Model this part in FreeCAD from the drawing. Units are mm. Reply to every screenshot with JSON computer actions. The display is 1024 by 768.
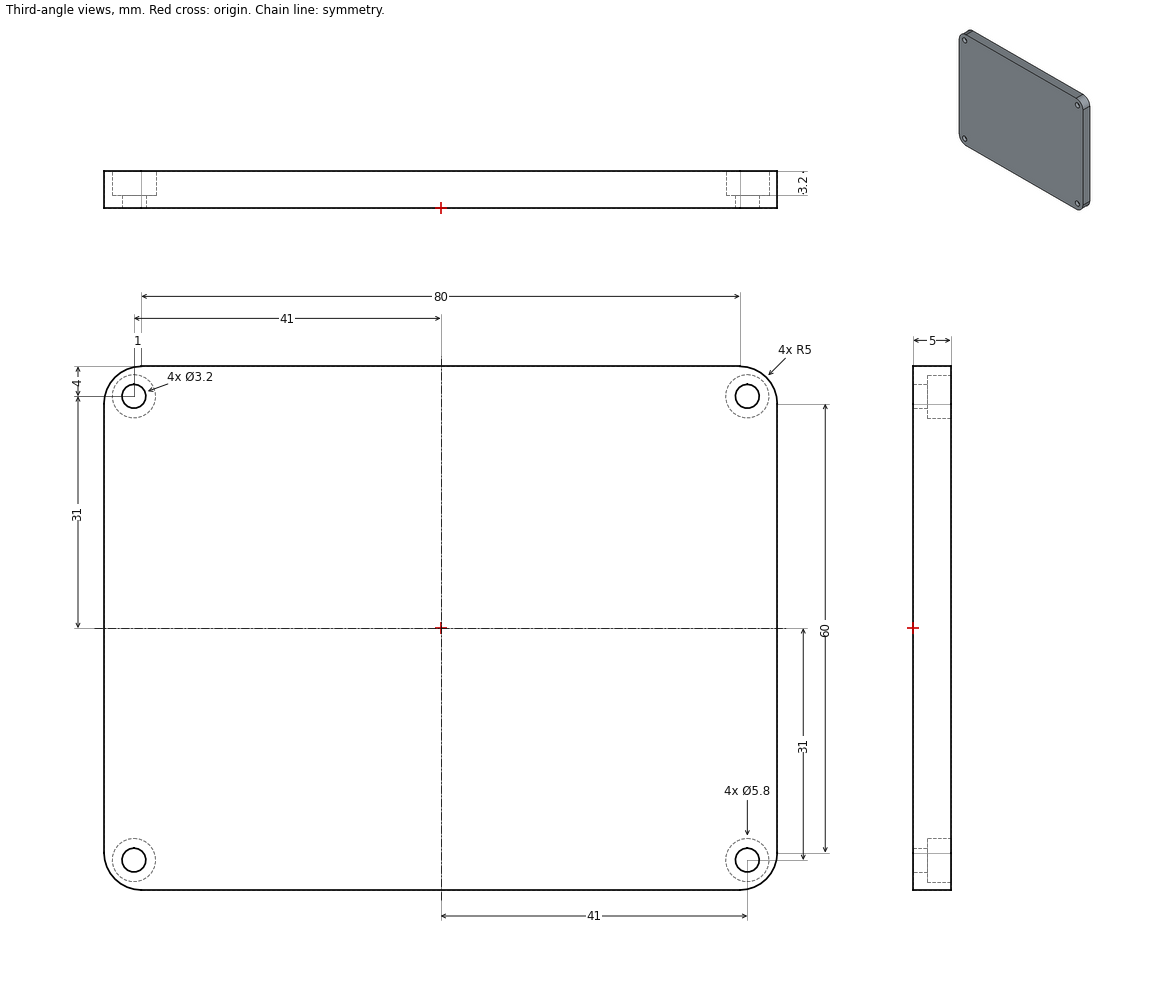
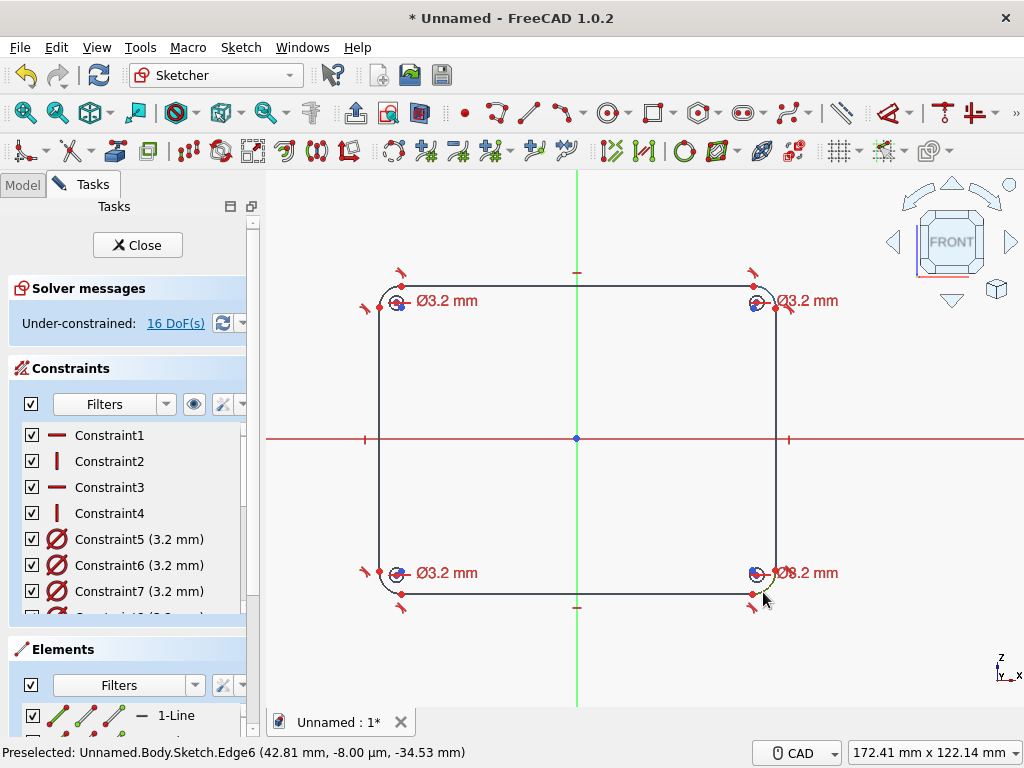
{"action": "scroll", "coordinate": [382, 582], "scroll_direction": "up", "scroll_amount": 3}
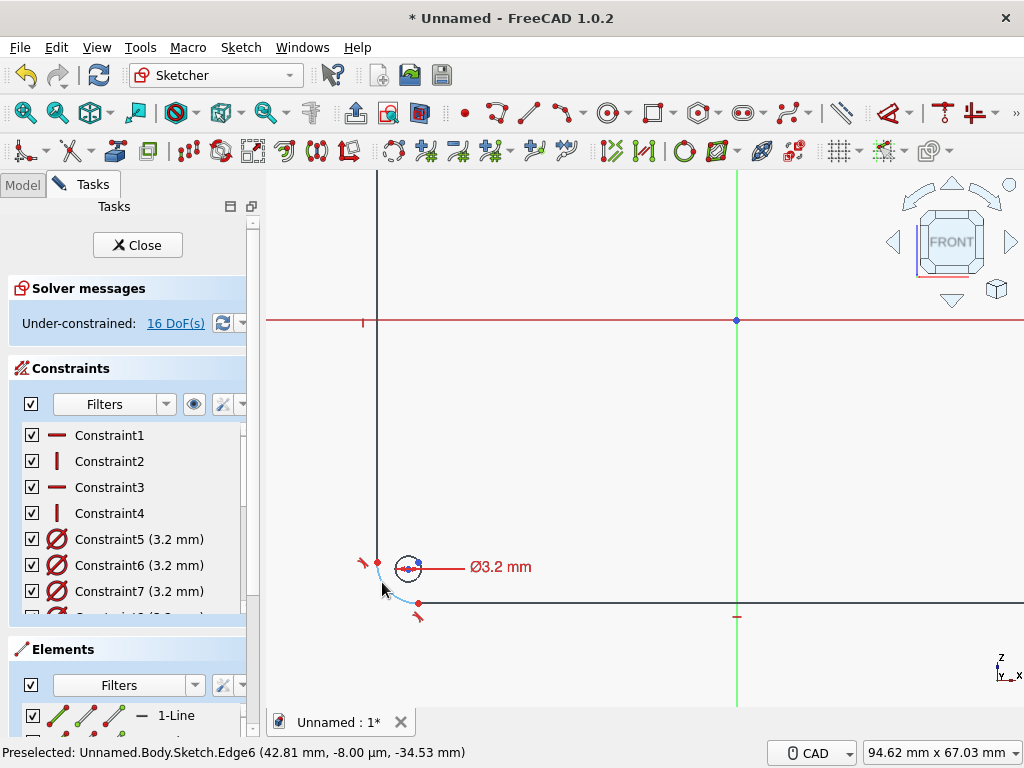
{"action": "left_click", "coordinate": [382, 581]}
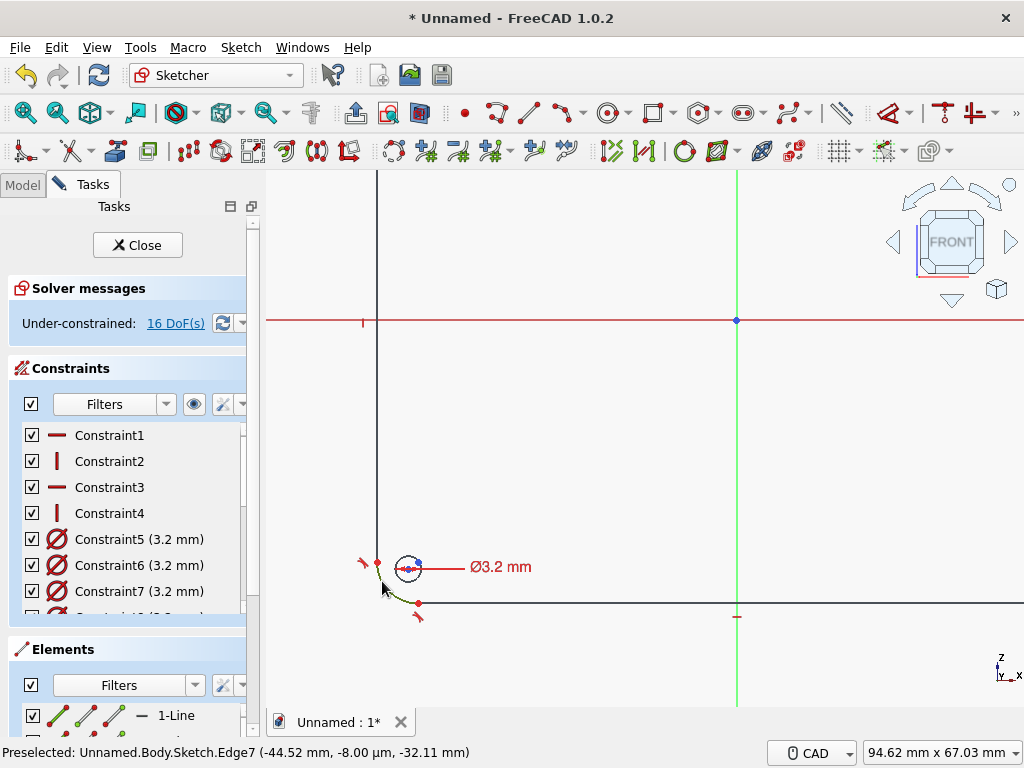
{"action": "scroll", "coordinate": [382, 582], "scroll_direction": "down", "scroll_amount": 3}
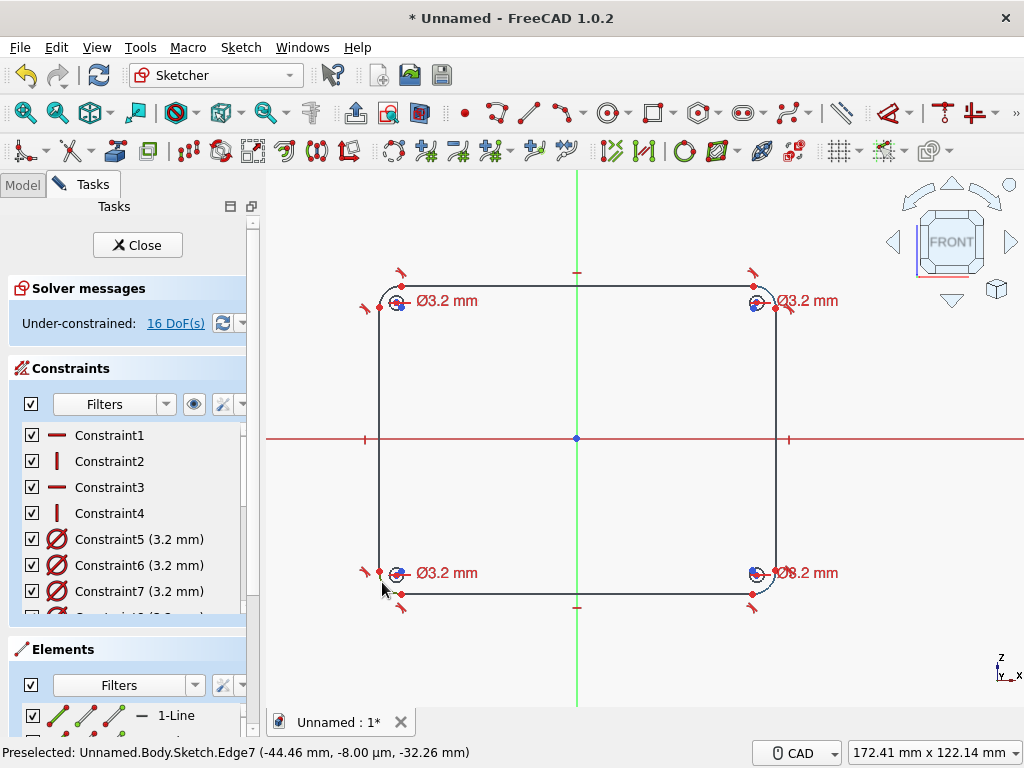
{"action": "scroll", "coordinate": [391, 288], "scroll_direction": "up", "scroll_amount": 3}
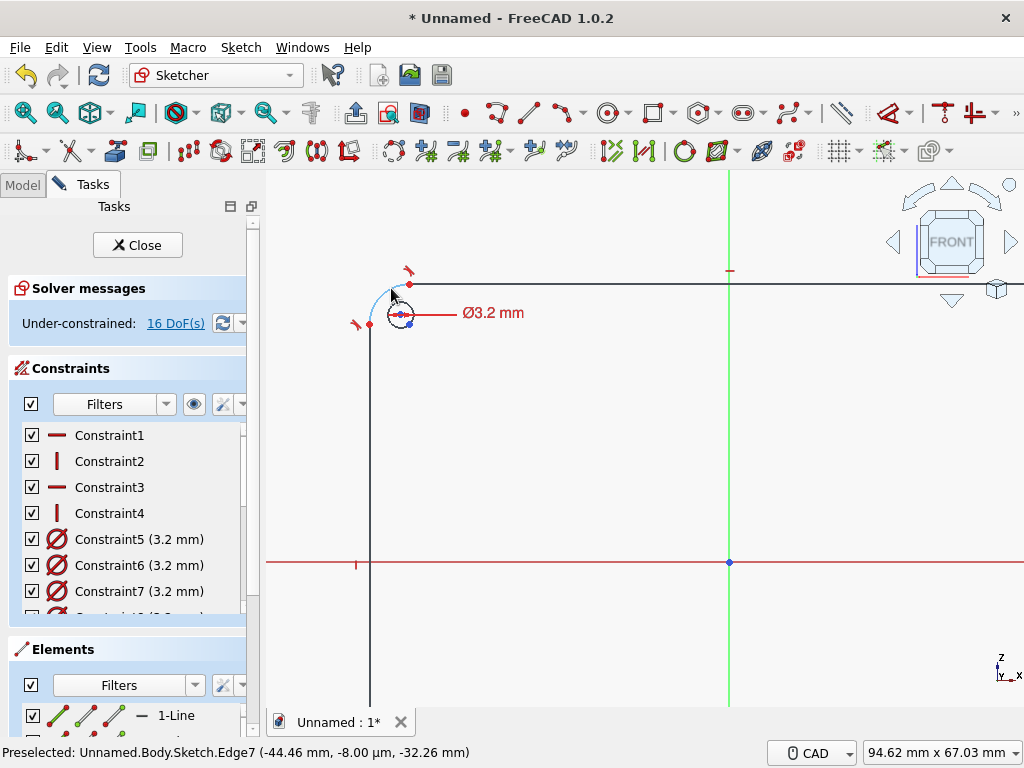
{"action": "left_click", "coordinate": [392, 289]}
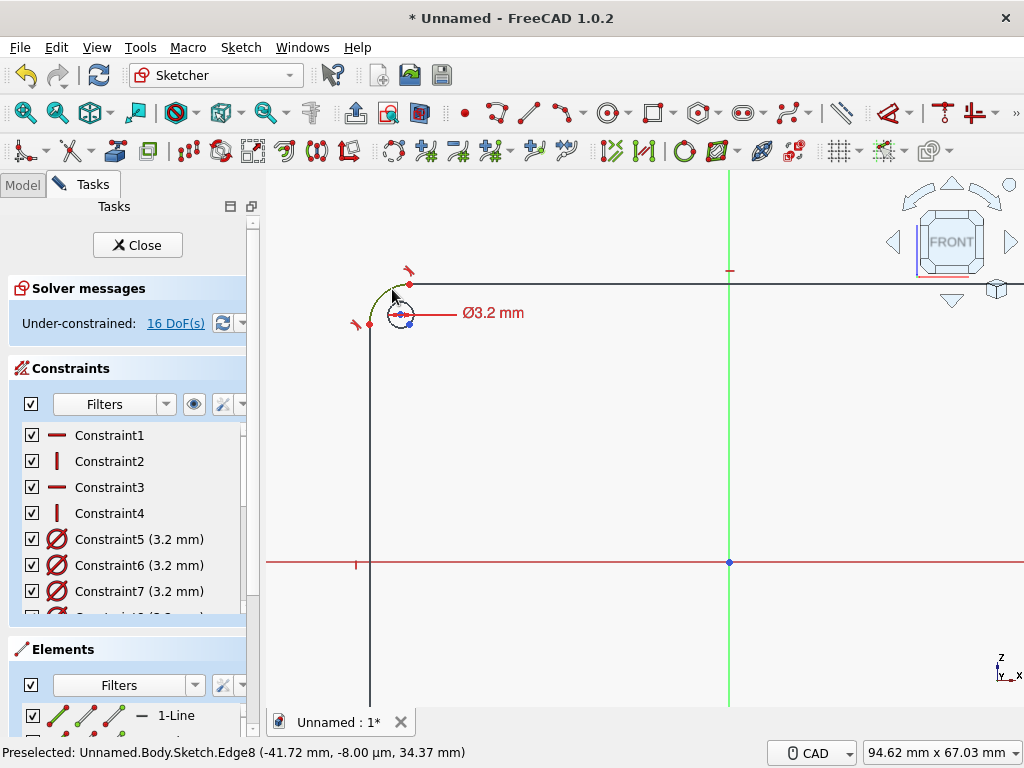
{"action": "key", "text": "e"}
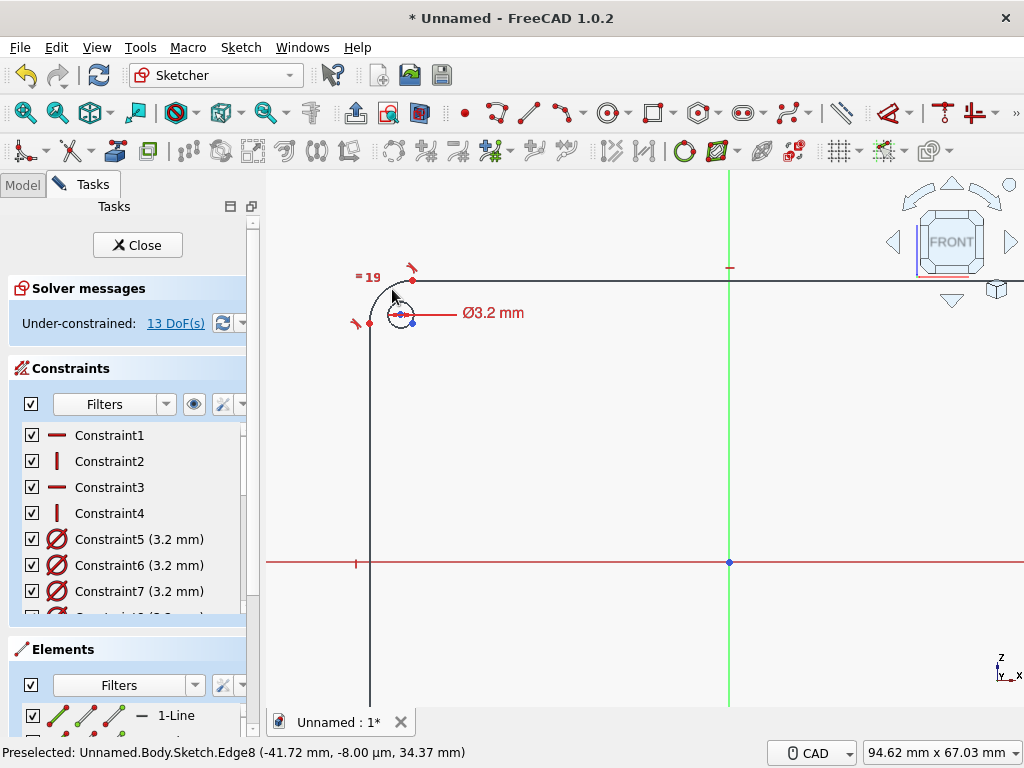
{"action": "left_click", "coordinate": [401, 315]}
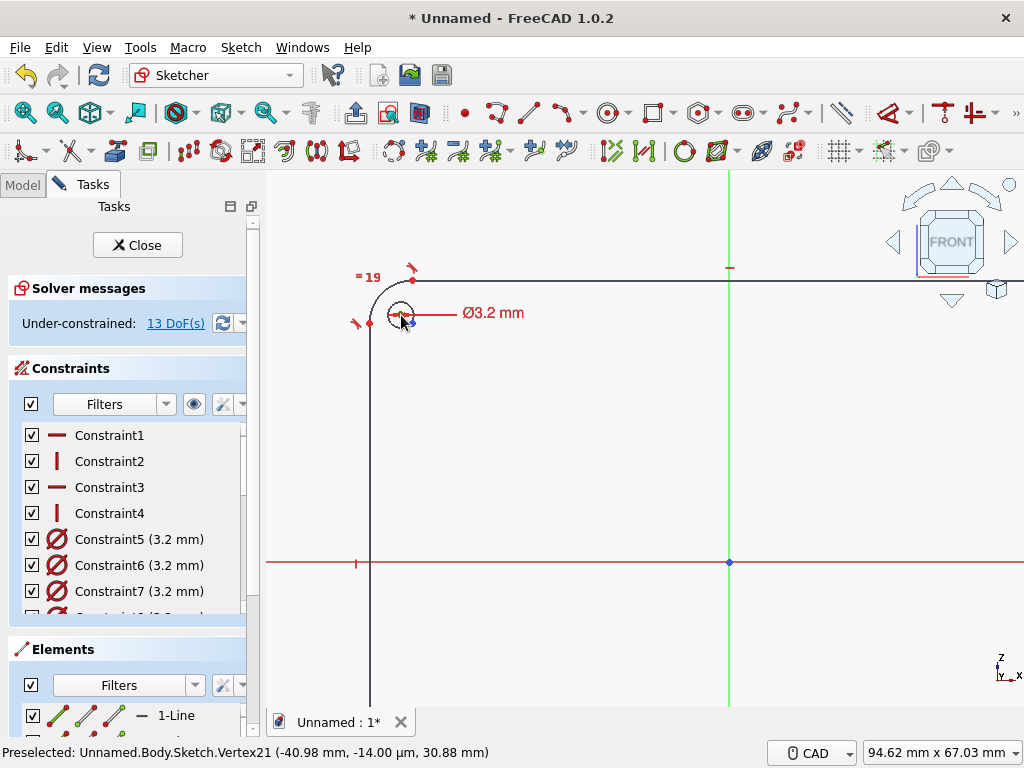
{"action": "scroll", "coordinate": [391, 288], "scroll_direction": "down", "scroll_amount": 3}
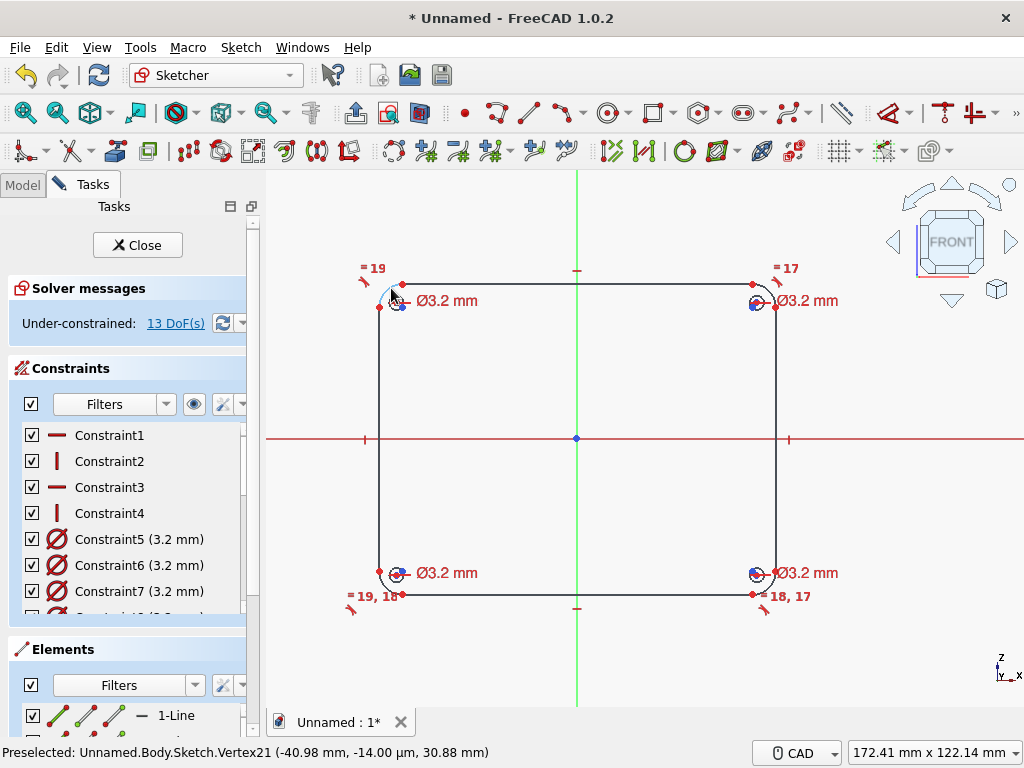
{"action": "scroll", "coordinate": [757, 303], "scroll_direction": "up", "scroll_amount": 4}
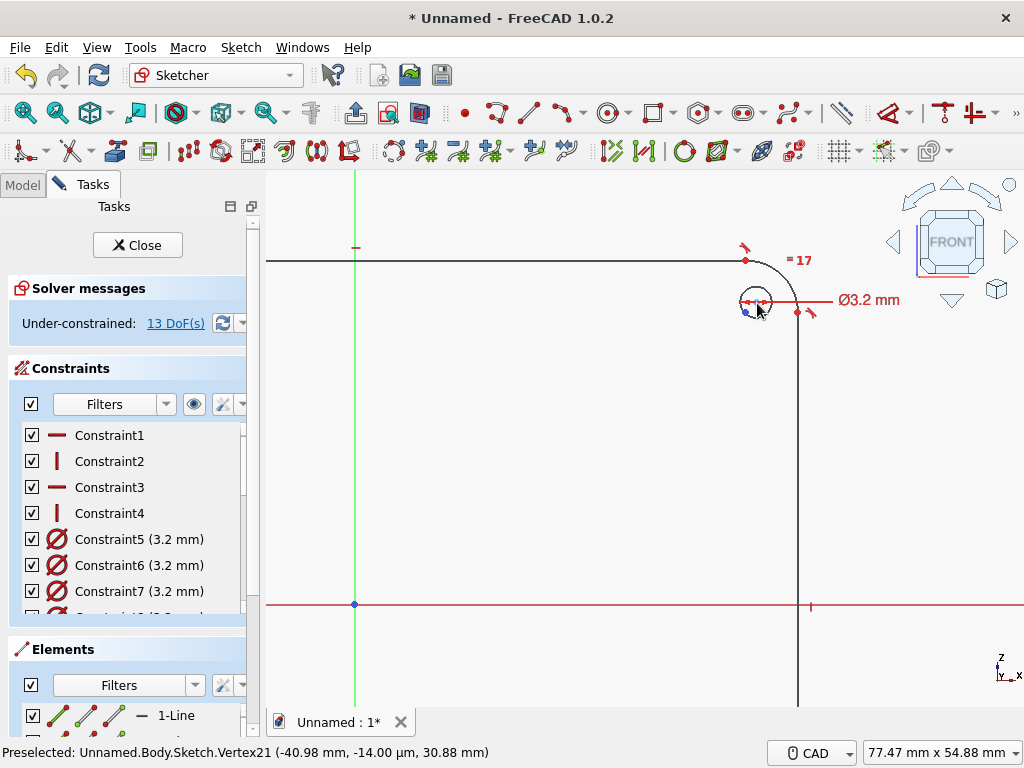
{"action": "left_click", "coordinate": [756, 302]}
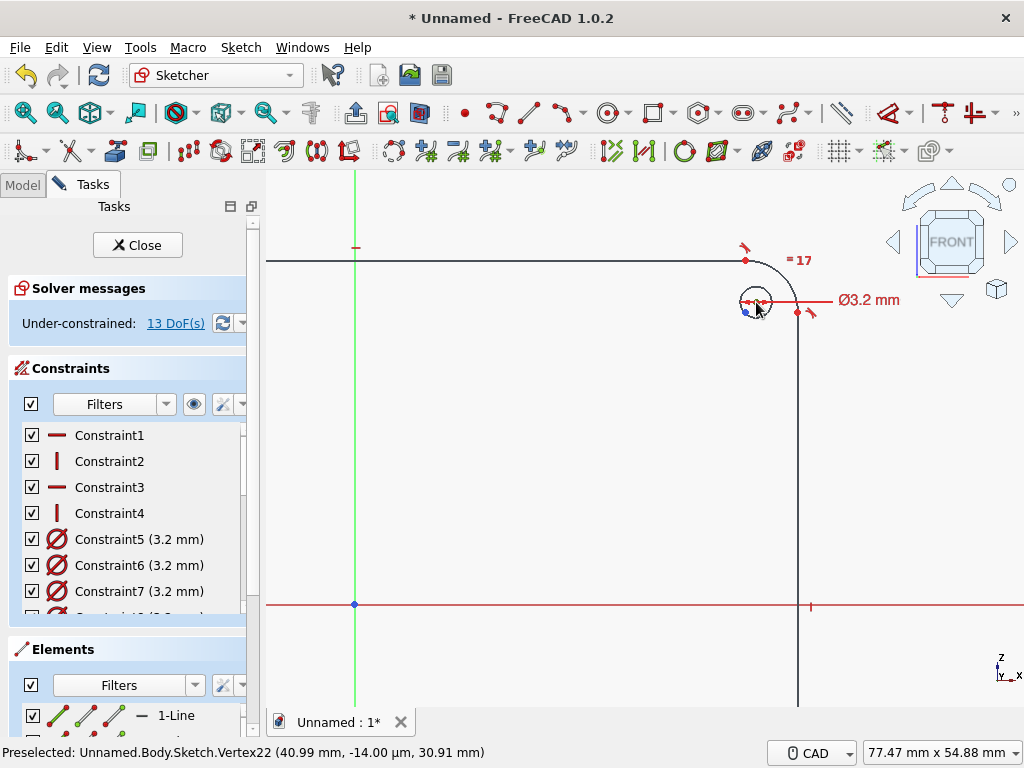
{"action": "left_click", "coordinate": [355, 645]}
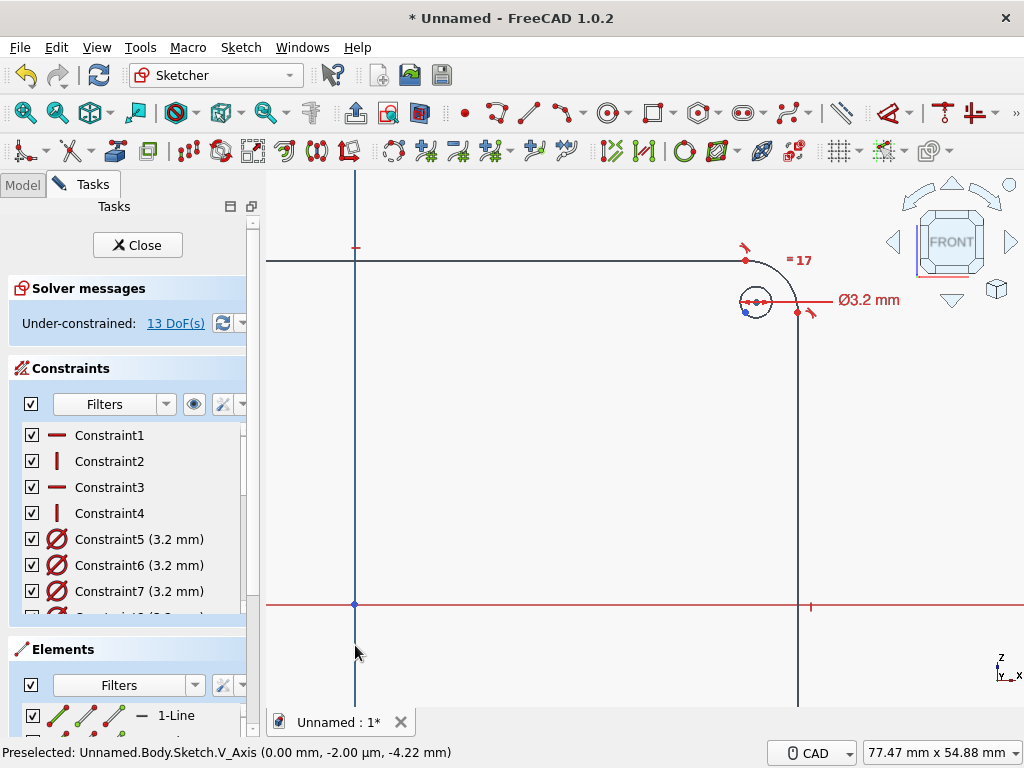
{"action": "key", "text": "s"}